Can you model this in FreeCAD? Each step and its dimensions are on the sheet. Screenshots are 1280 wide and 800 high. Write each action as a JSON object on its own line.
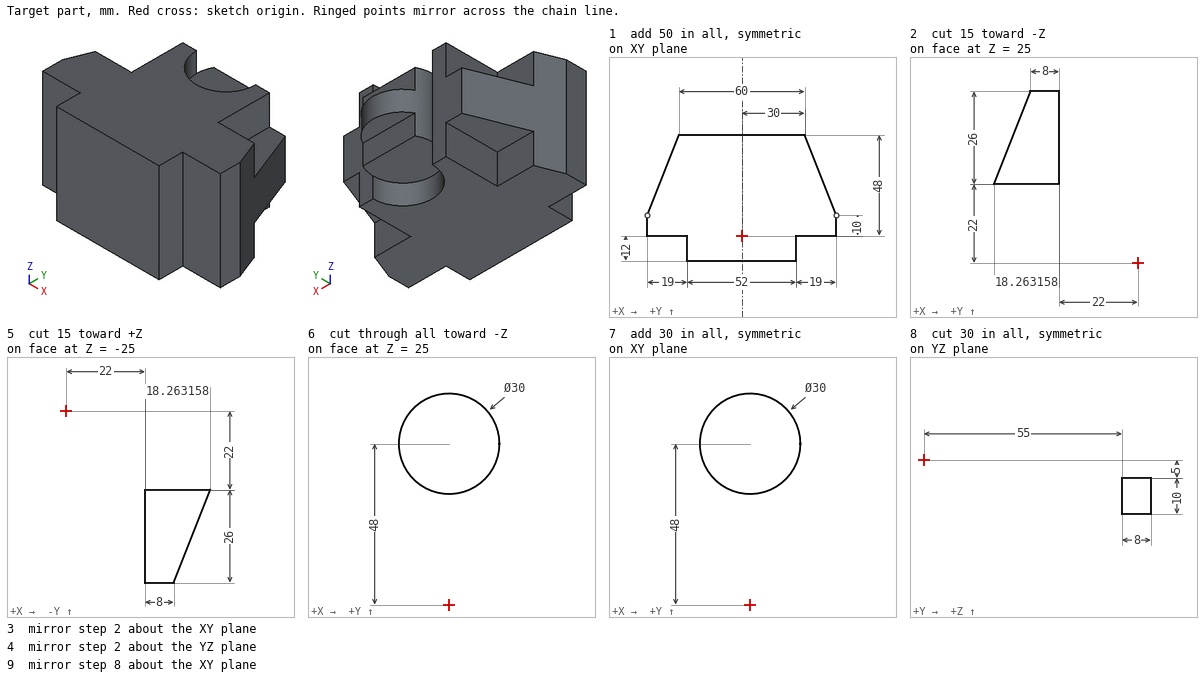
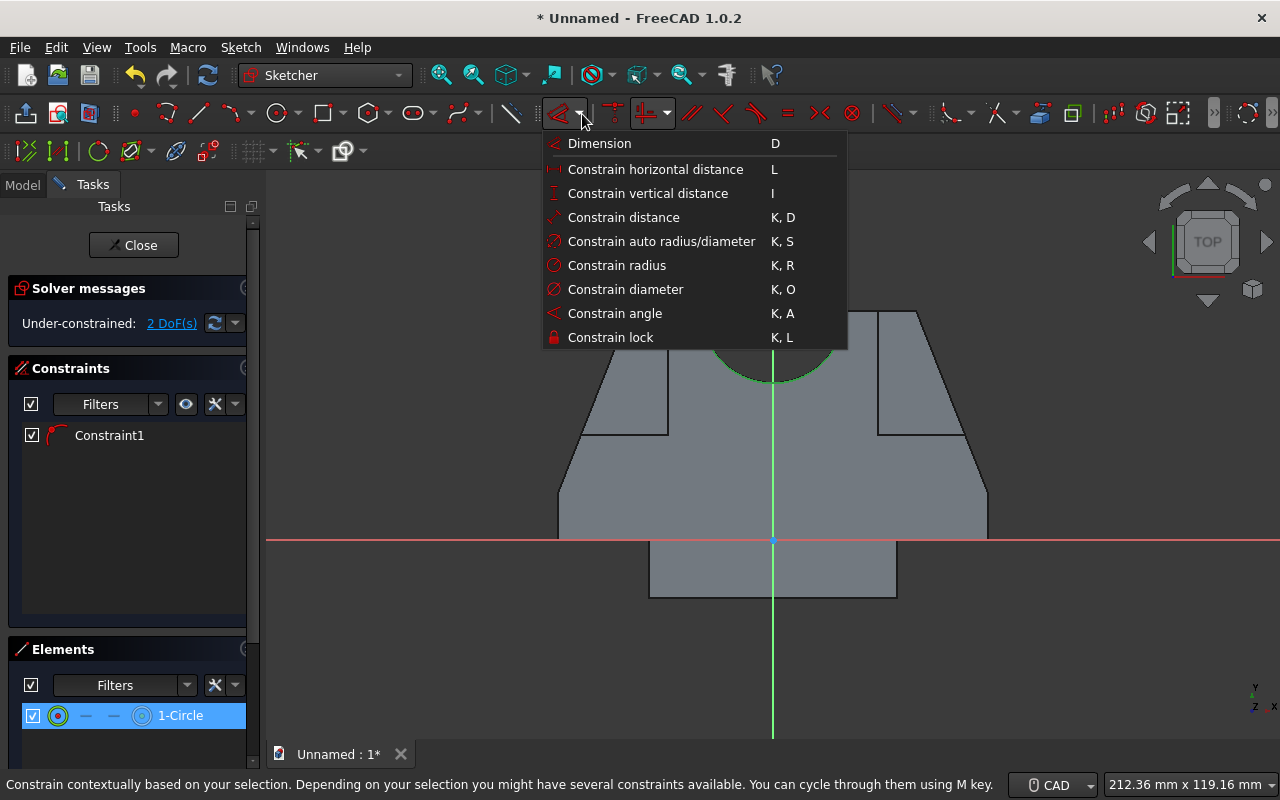
{"action": "left_click", "coordinate": [695, 289]}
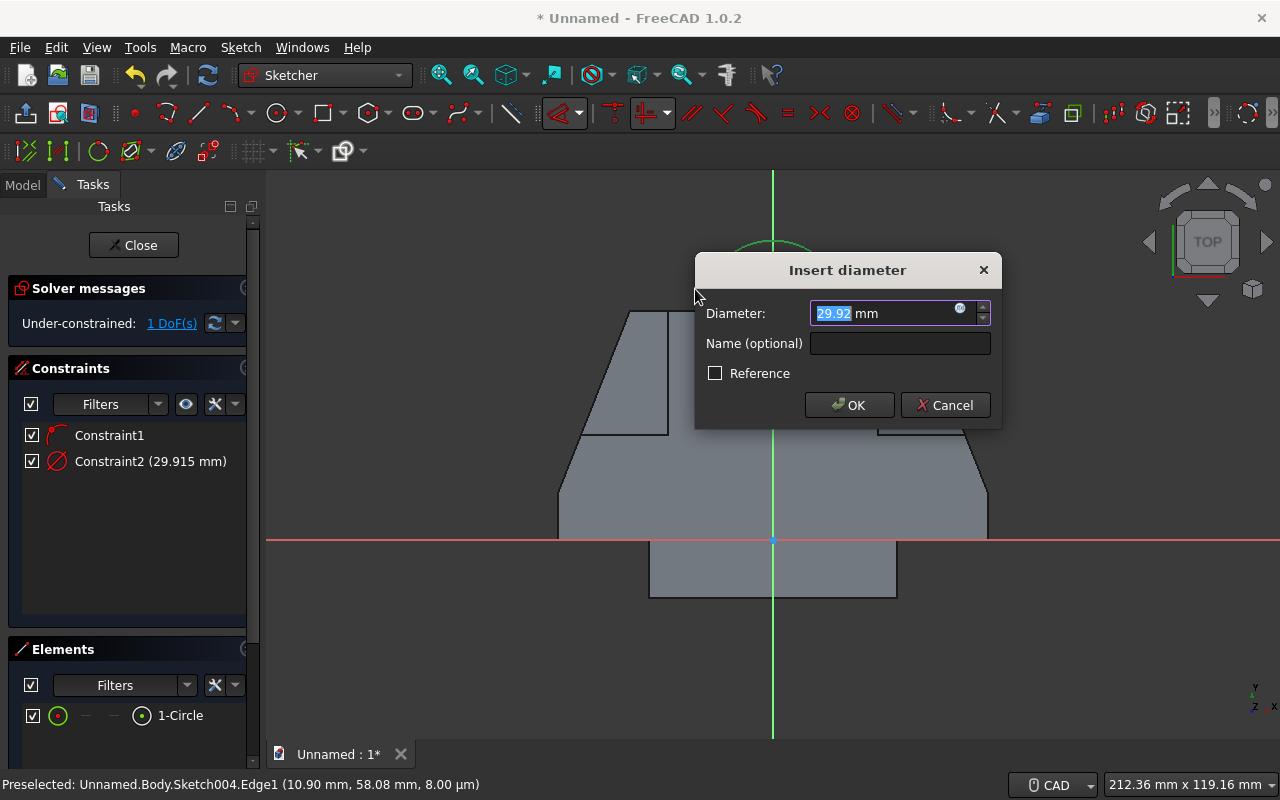
{"action": "type", "text": "30"}
{"action": "key", "text": "Return"}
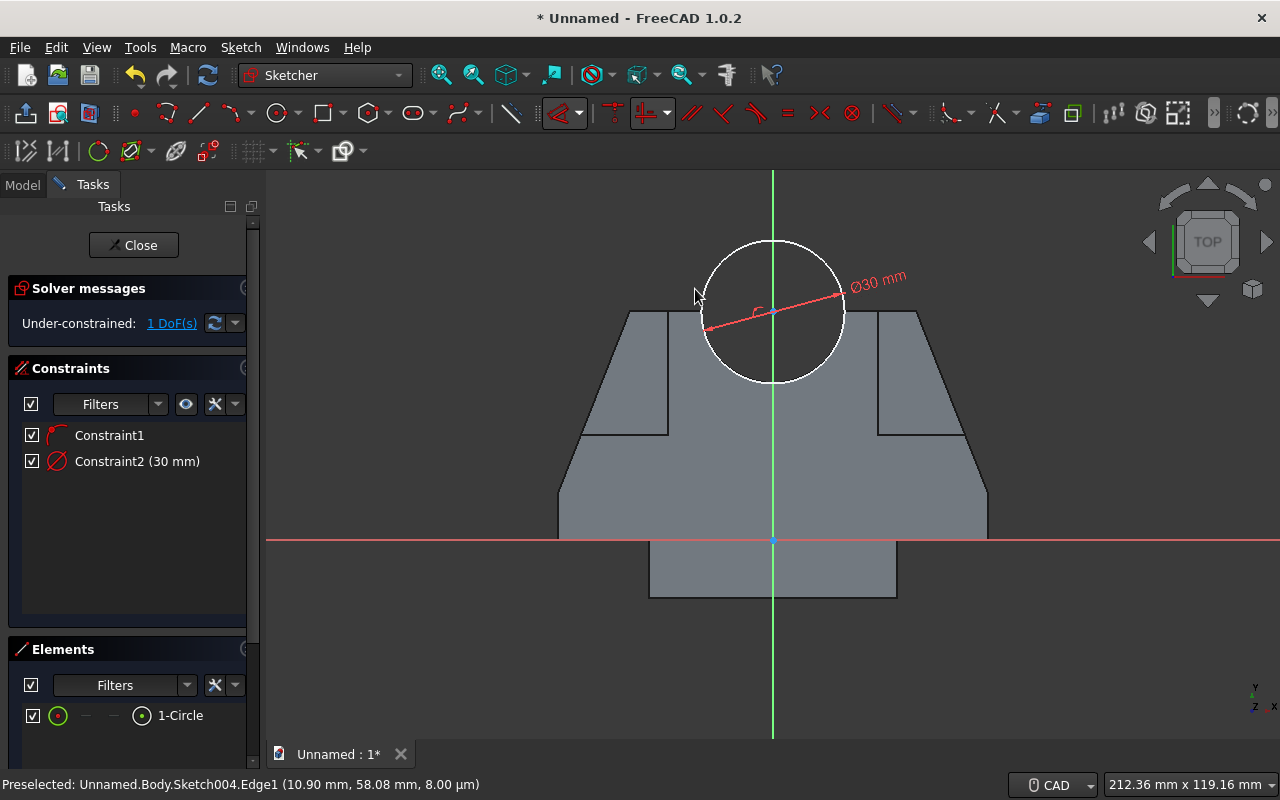
{"action": "left_click", "coordinate": [773, 312]}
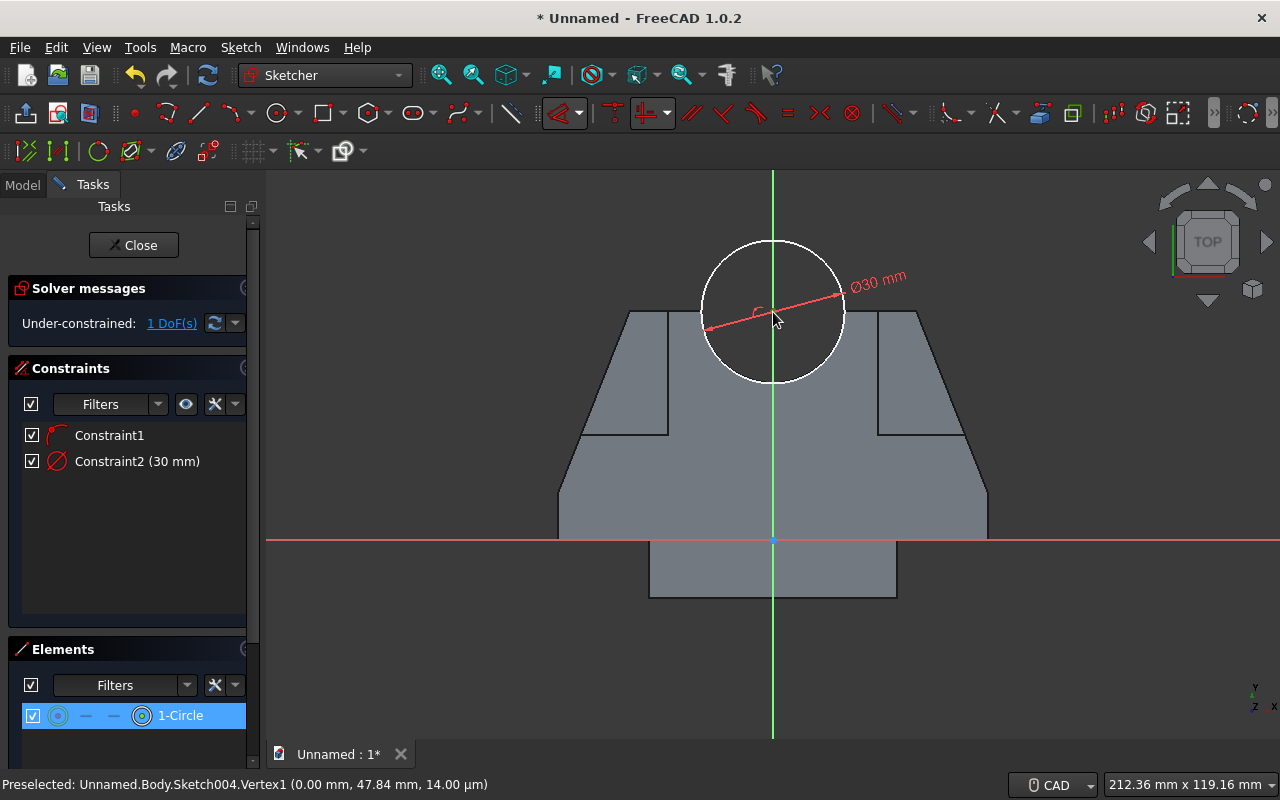
{"action": "left_click", "coordinate": [582, 114]}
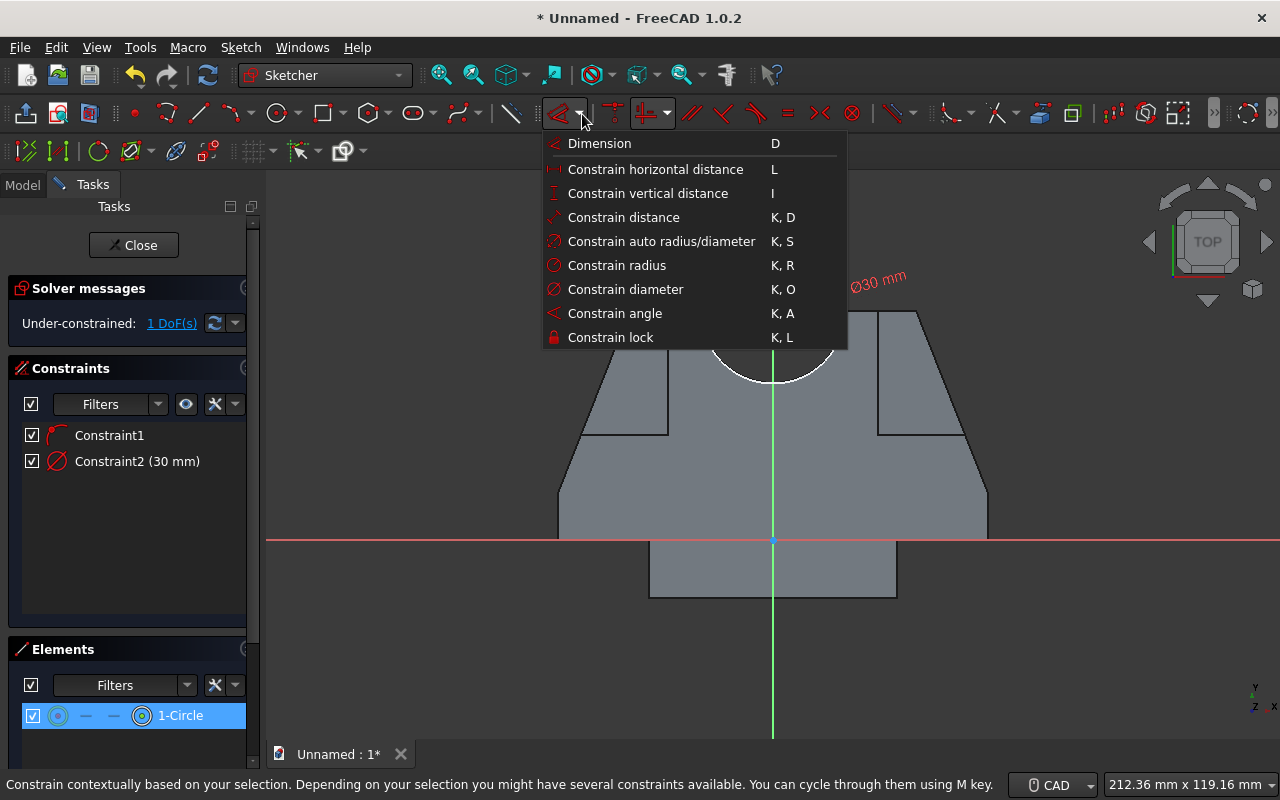
{"action": "left_click", "coordinate": [695, 193]}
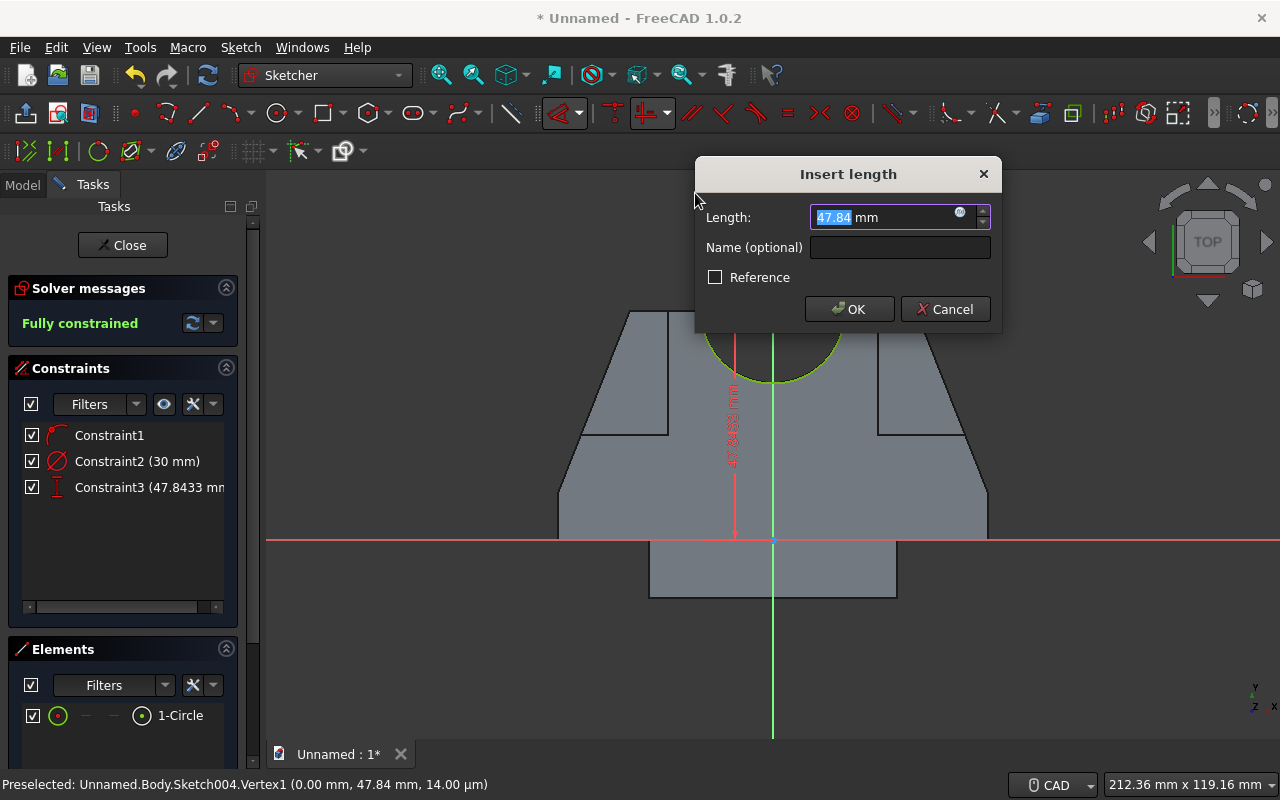
{"action": "type", "text": "48"}
{"action": "key", "text": "Return"}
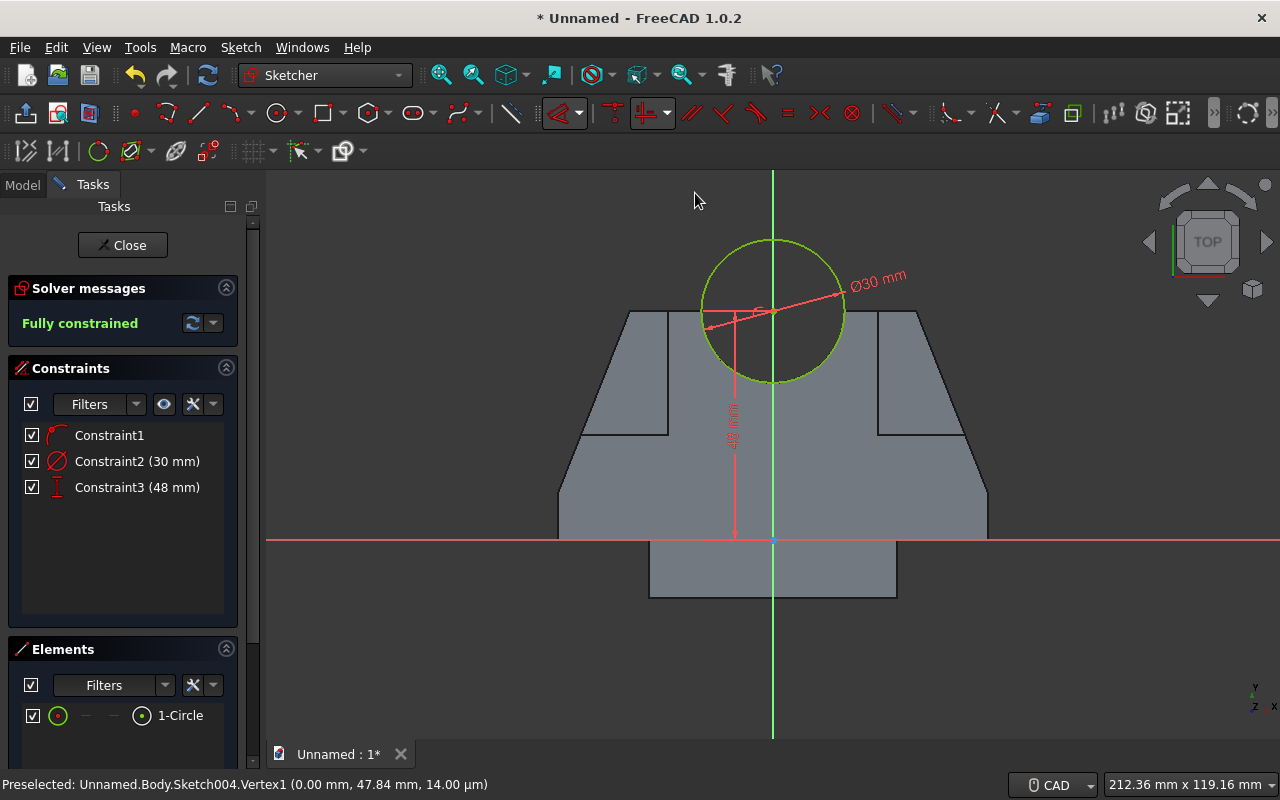
{"action": "left_click", "coordinate": [123, 245]}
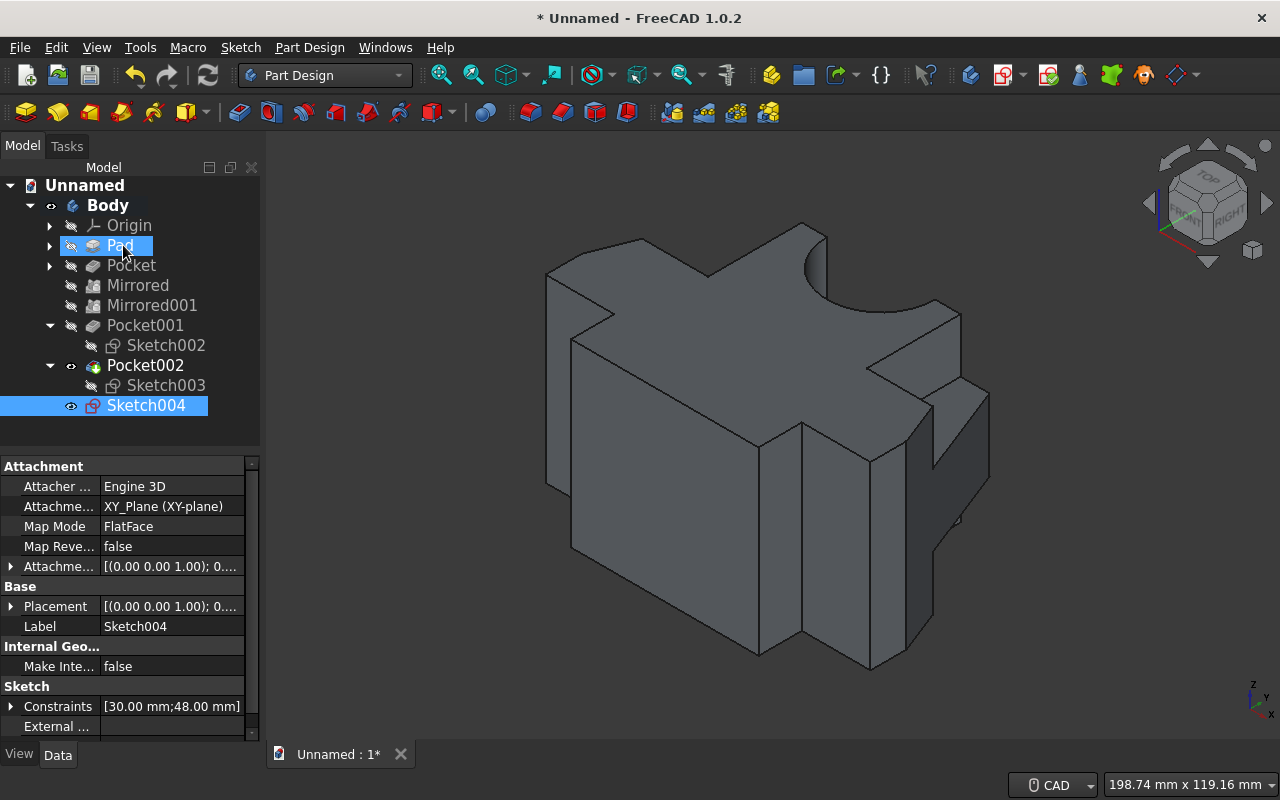
{"action": "left_click", "coordinate": [26, 112]}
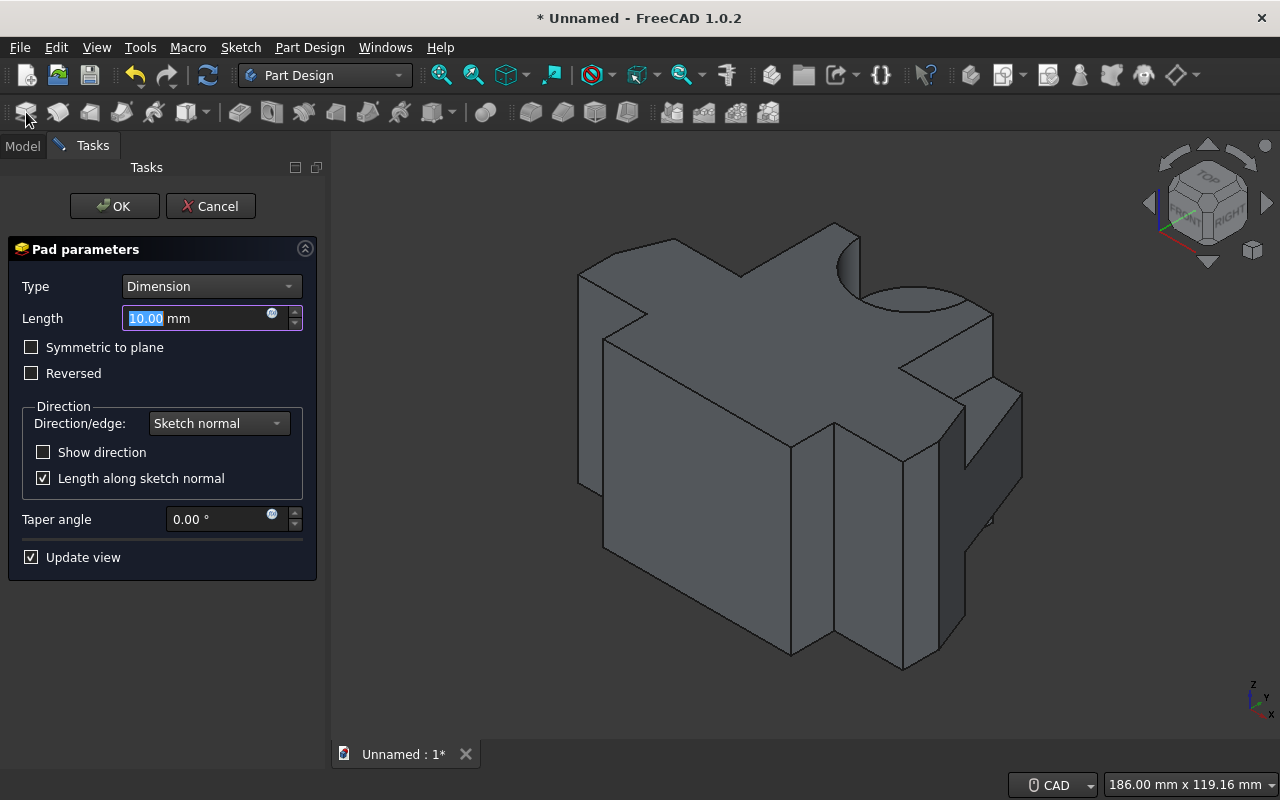
{"action": "type", "text": "30"}
{"action": "key", "text": "Tab"}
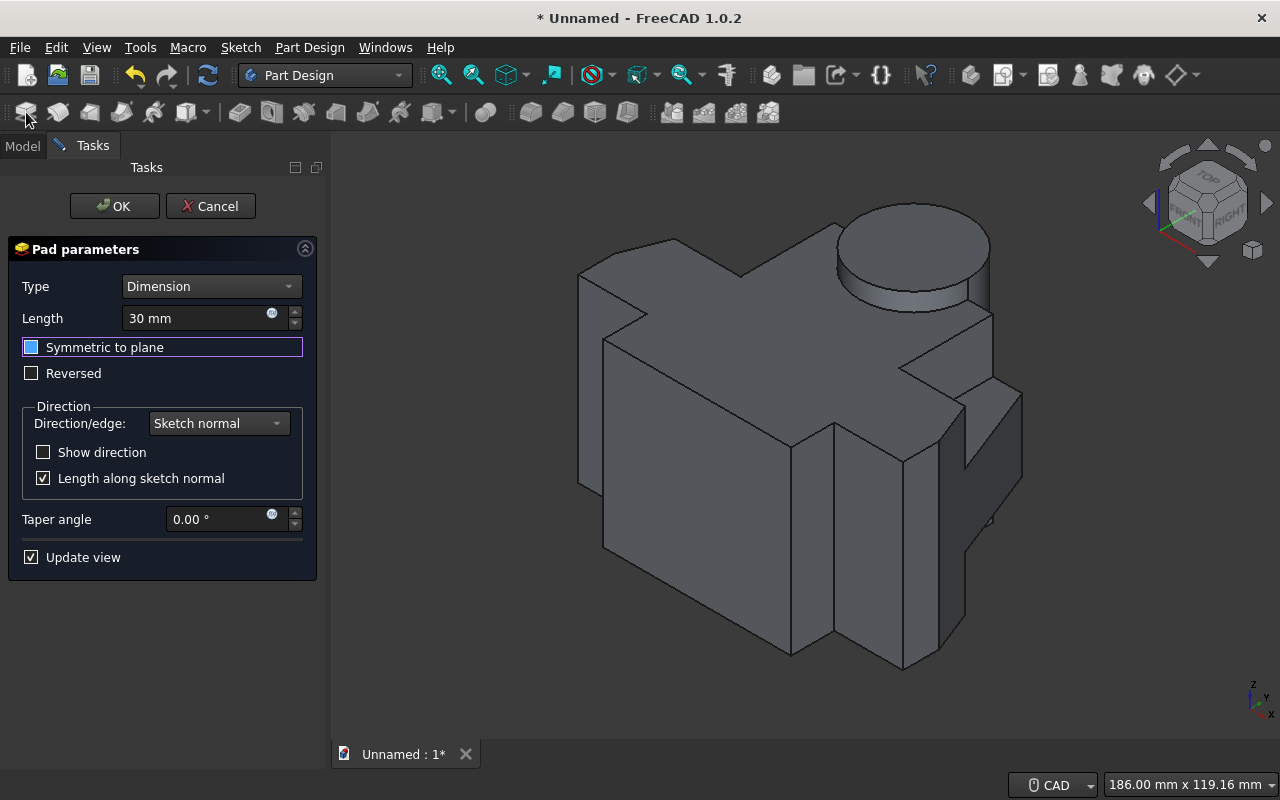
{"action": "left_click", "coordinate": [30, 347]}